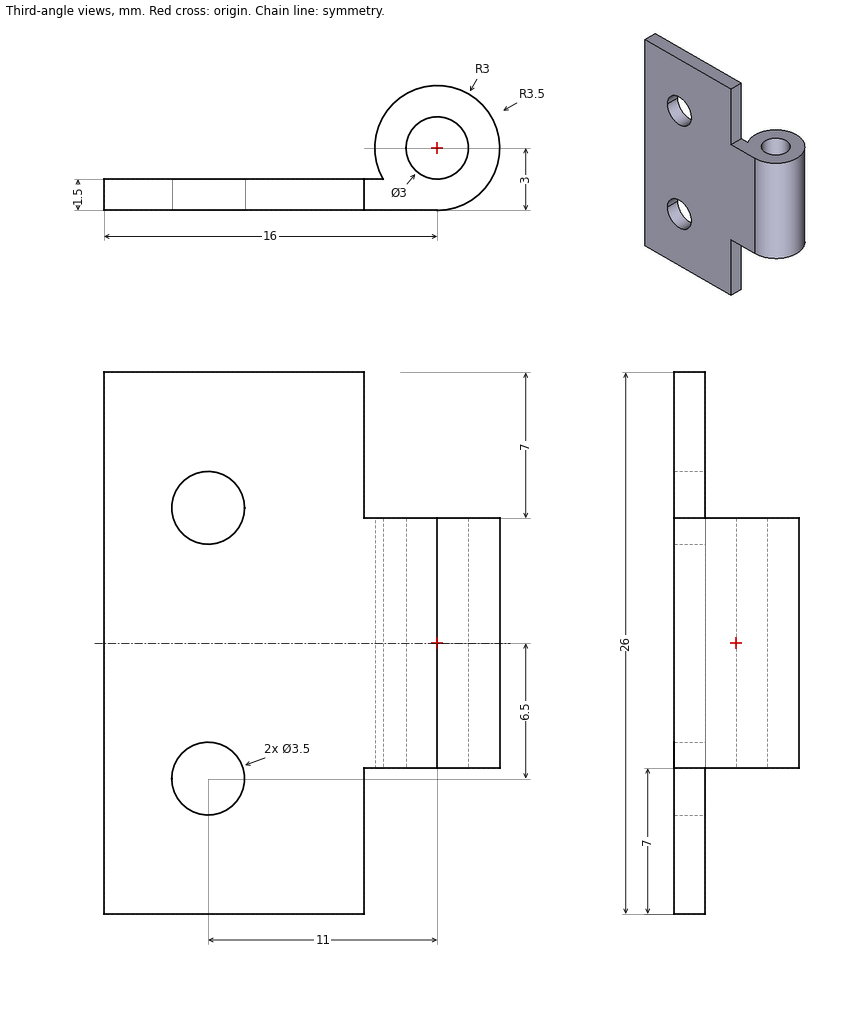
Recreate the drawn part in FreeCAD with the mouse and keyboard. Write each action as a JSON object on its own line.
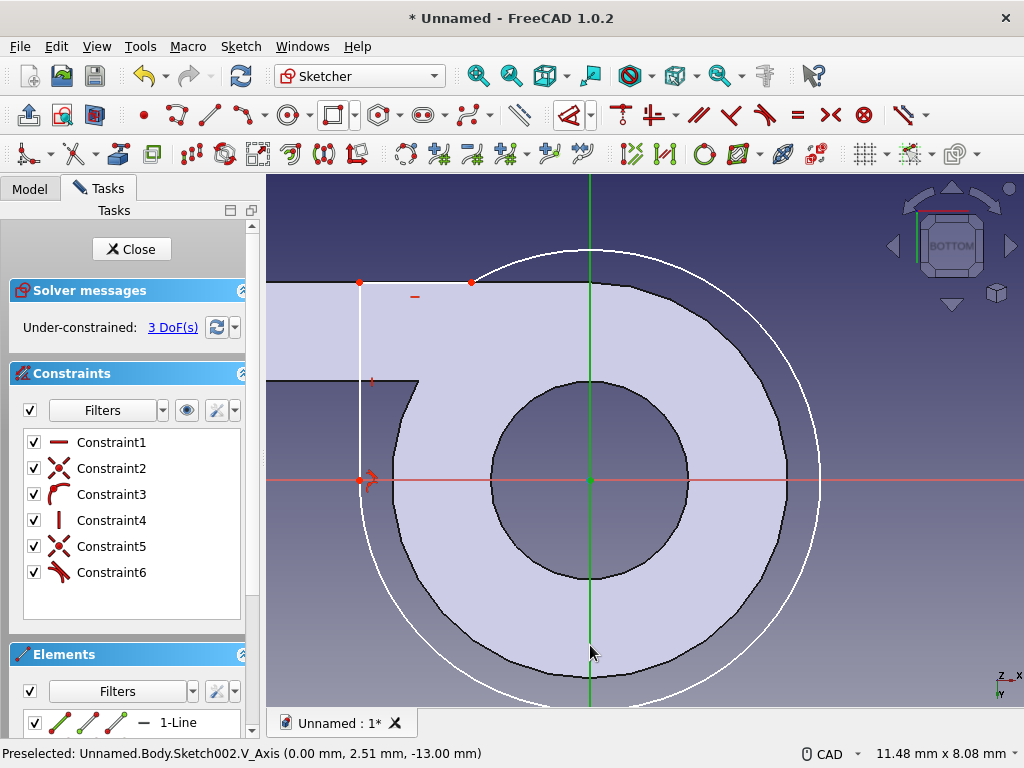
{"action": "key", "text": "c"}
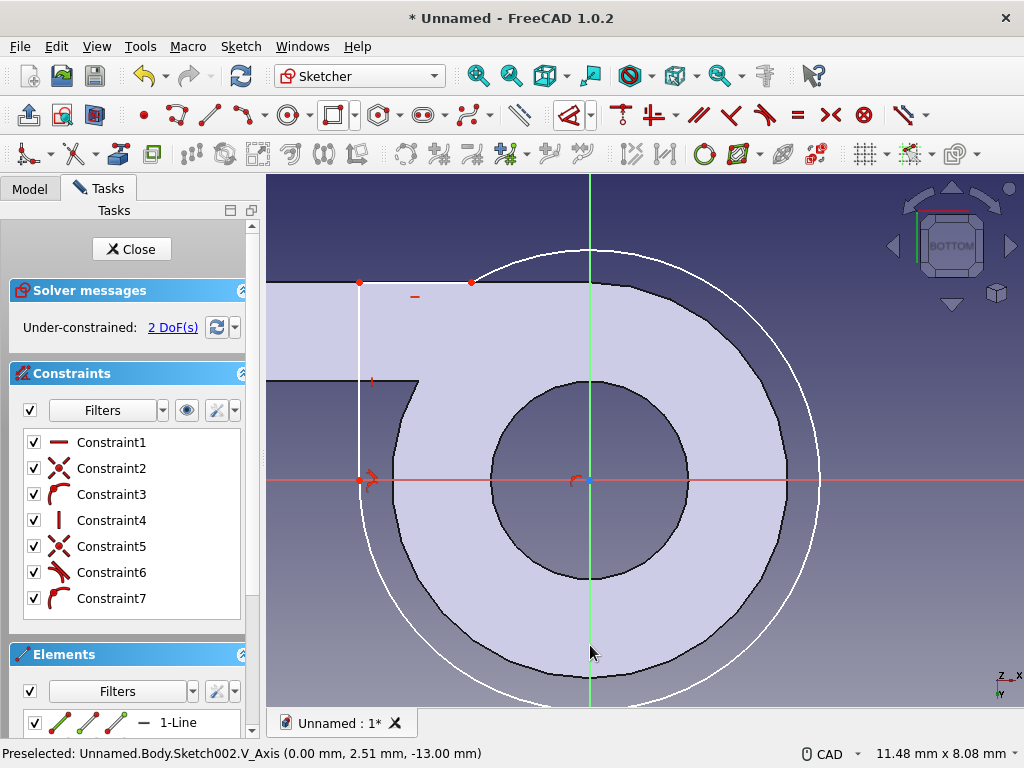
{"action": "left_click", "coordinate": [788, 363]}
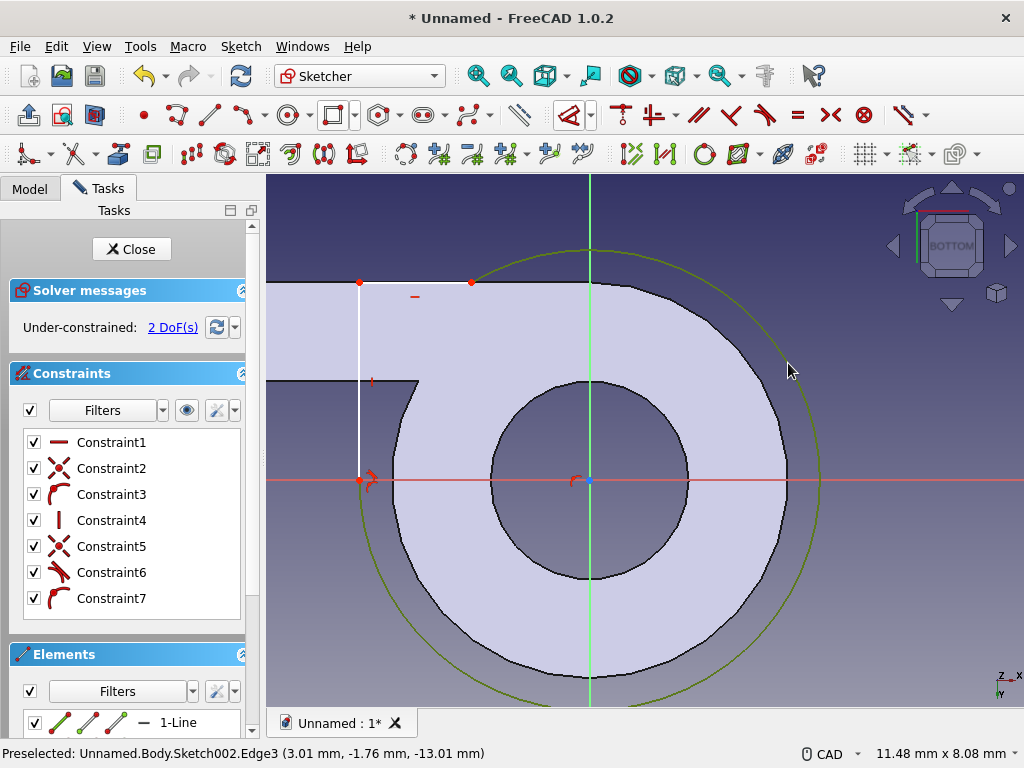
{"action": "key", "text": "k r"}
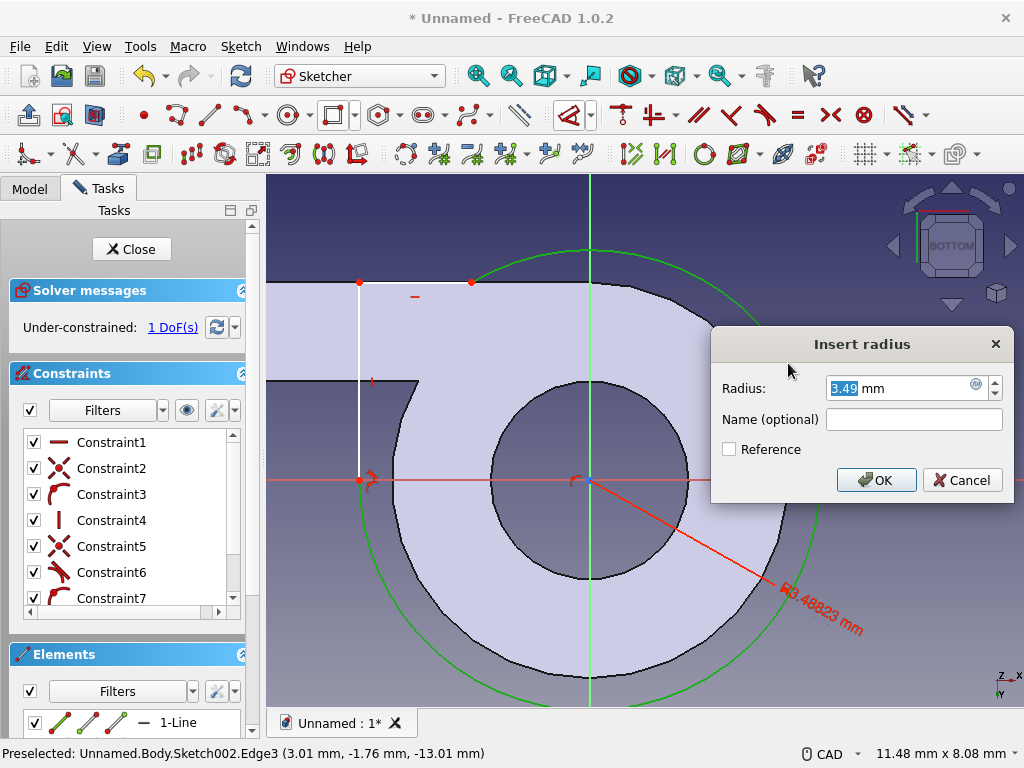
{"action": "type", "text": "3.5"}
{"action": "key", "text": "Return"}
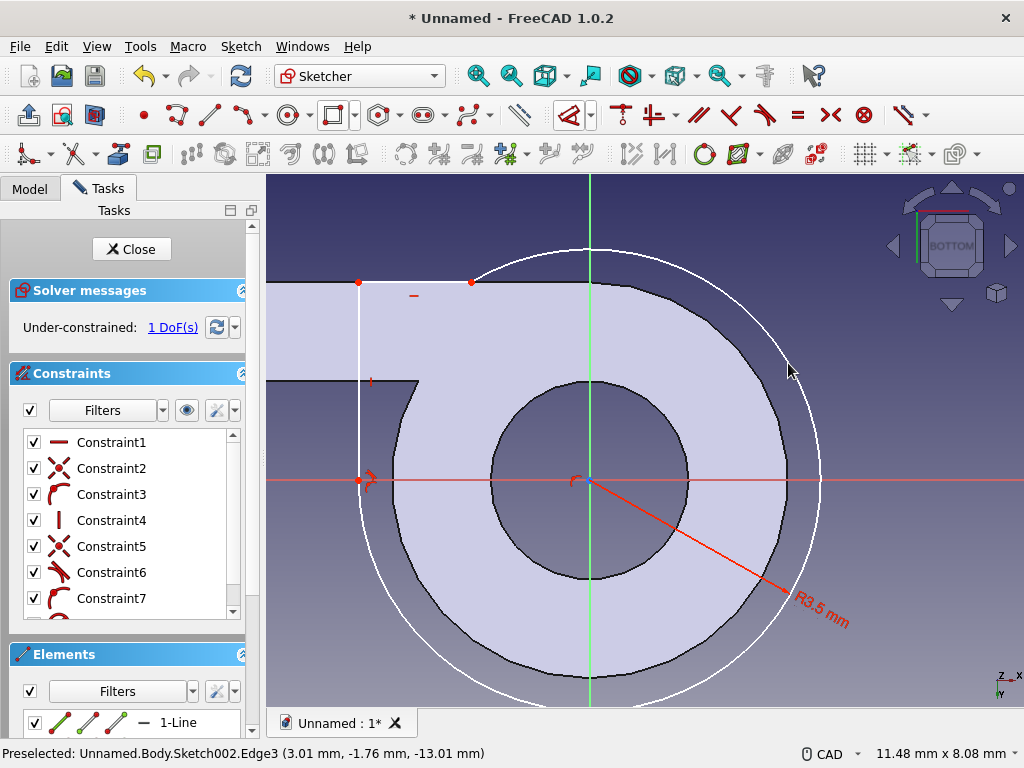
{"action": "left_click", "coordinate": [359, 342]}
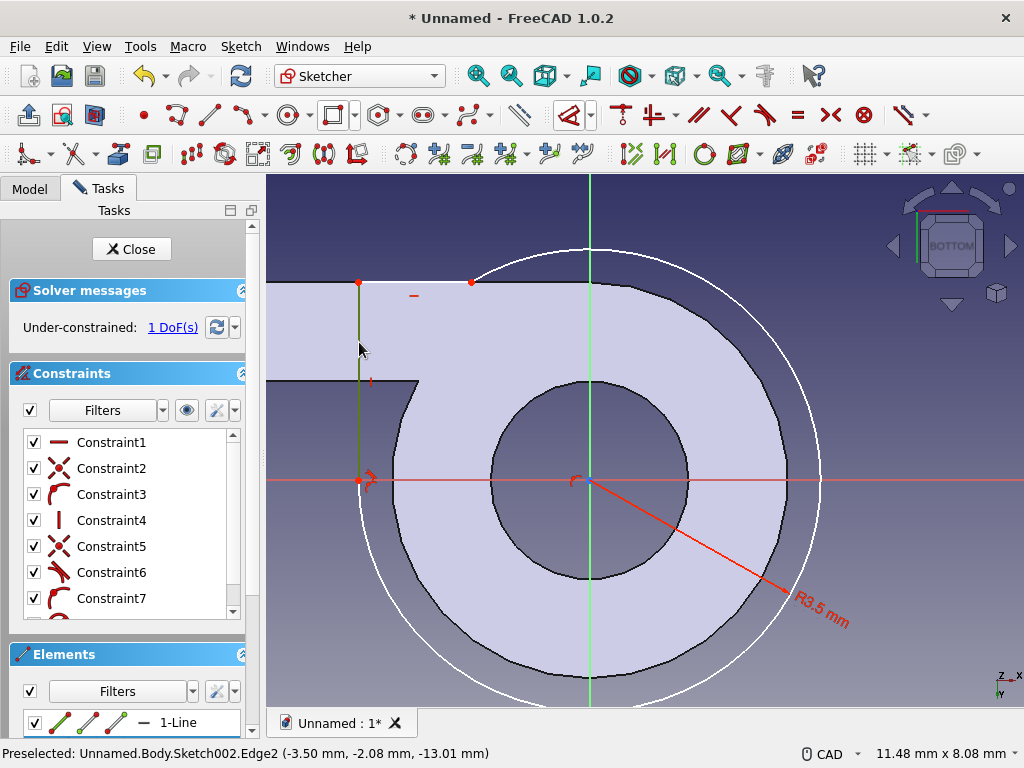
{"action": "key", "text": "i"}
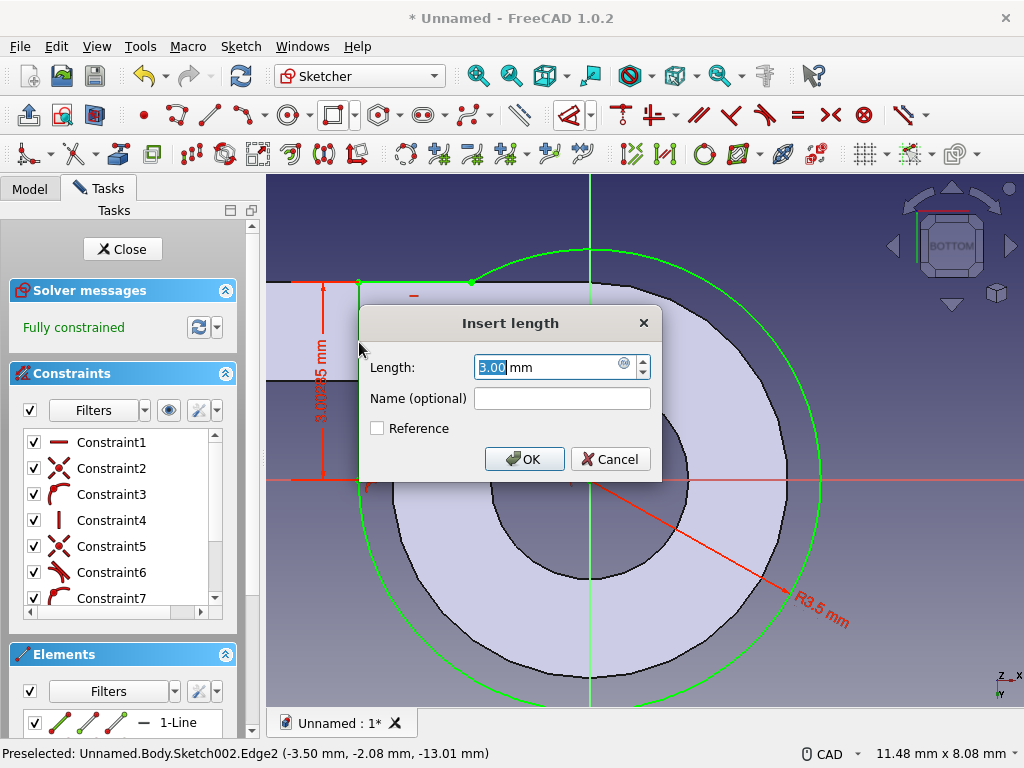
{"action": "type", "text": "3"}
{"action": "key", "text": "Return"}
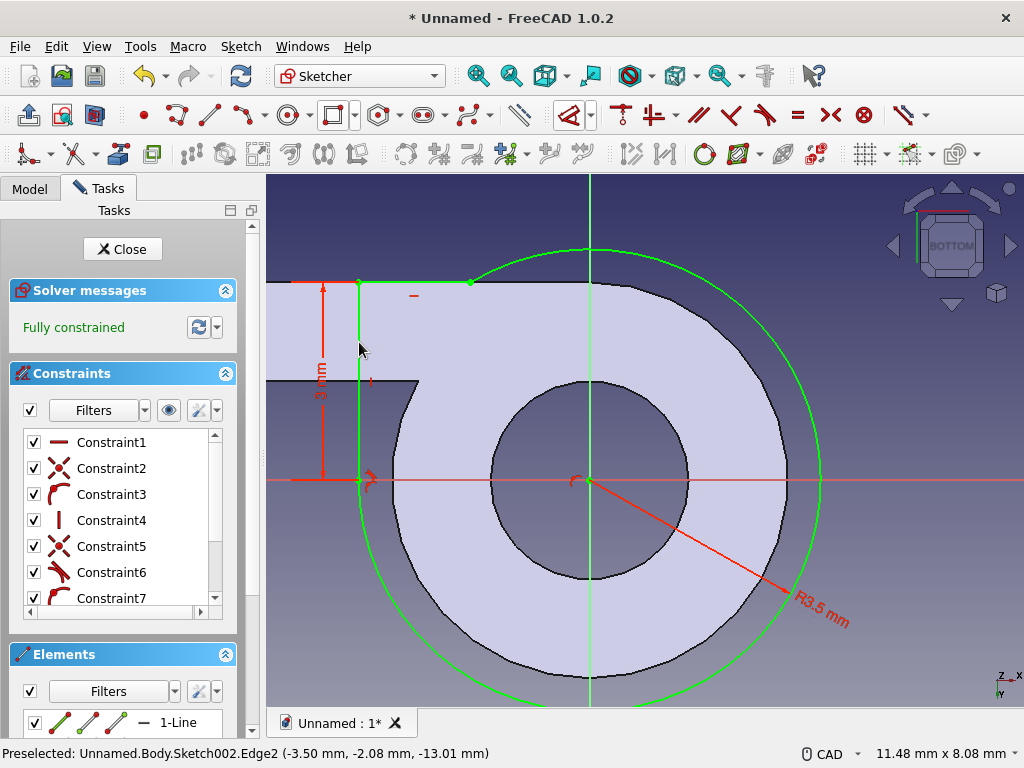
{"action": "left_click", "coordinate": [123, 249]}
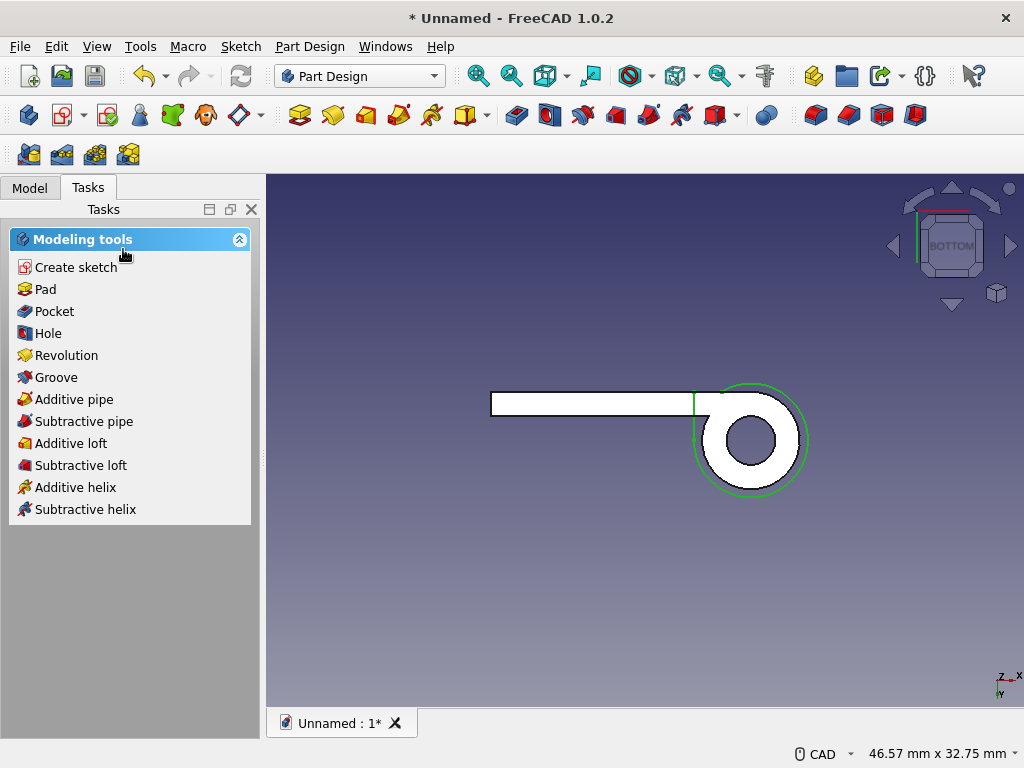
{"action": "left_click", "coordinate": [517, 116]}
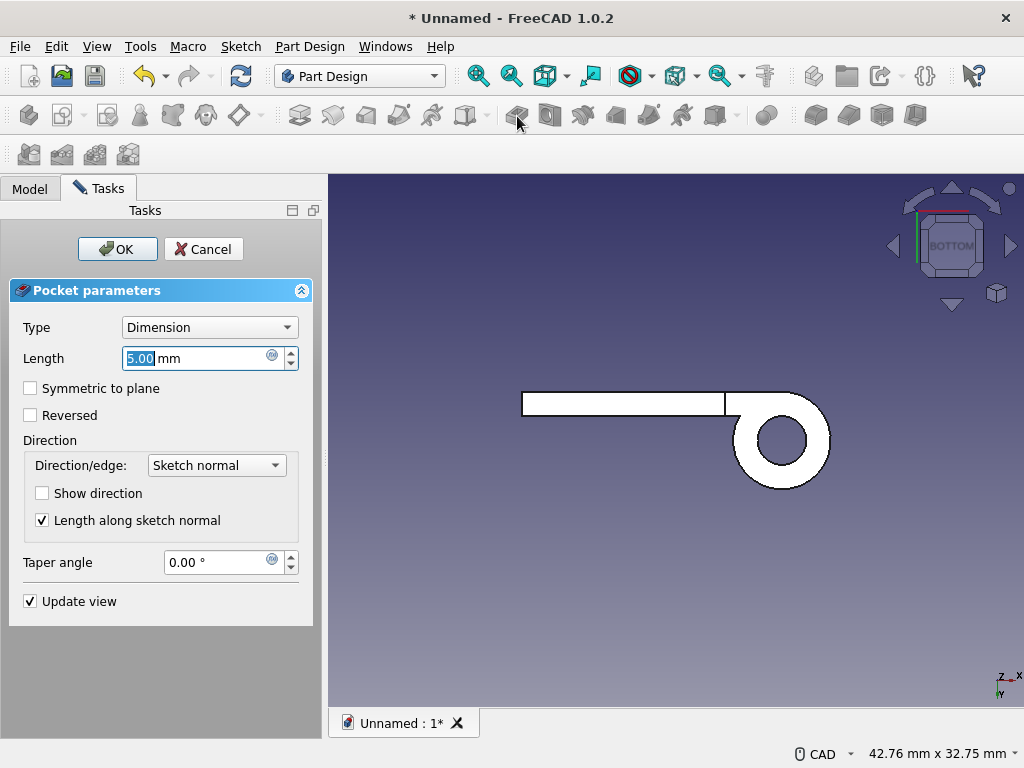
{"action": "type", "text": "7"}
{"action": "key", "text": "Tab"}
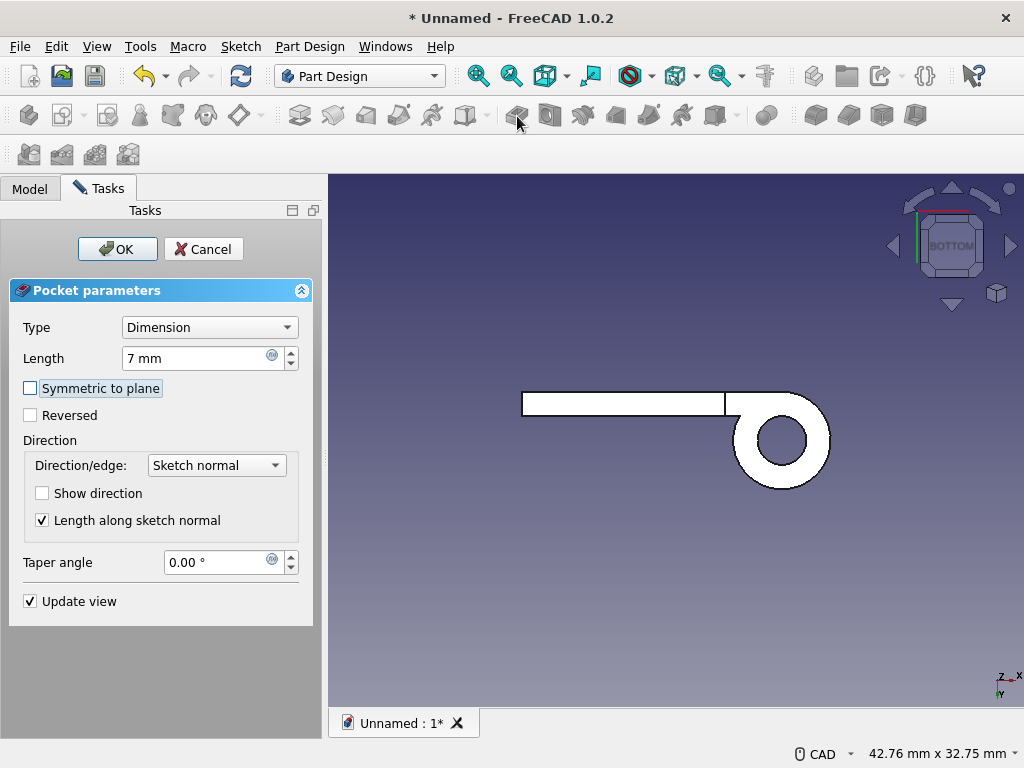
{"action": "left_click", "coordinate": [118, 249]}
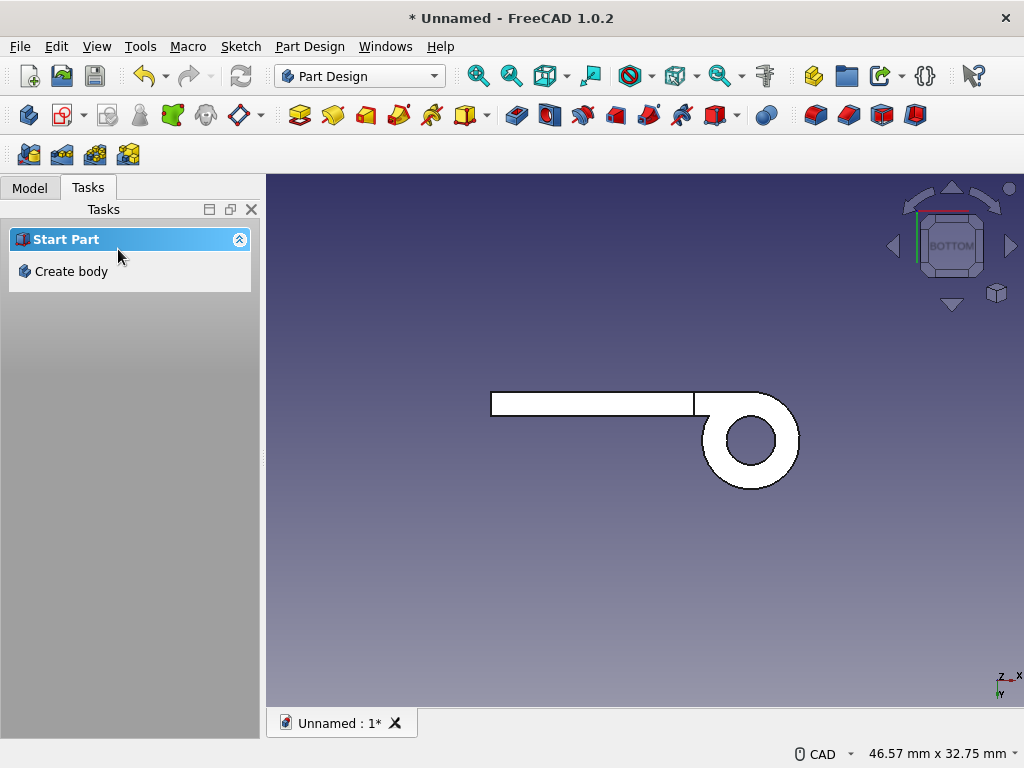
{"action": "key", "text": "v f"}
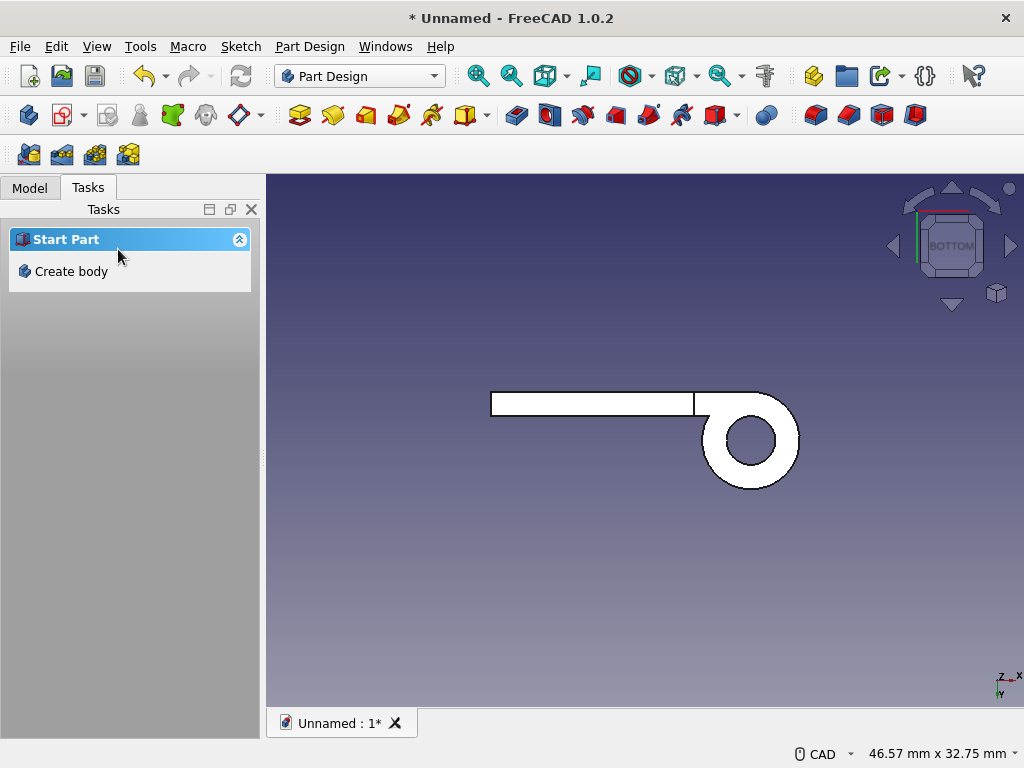
{"action": "key", "text": "4"}